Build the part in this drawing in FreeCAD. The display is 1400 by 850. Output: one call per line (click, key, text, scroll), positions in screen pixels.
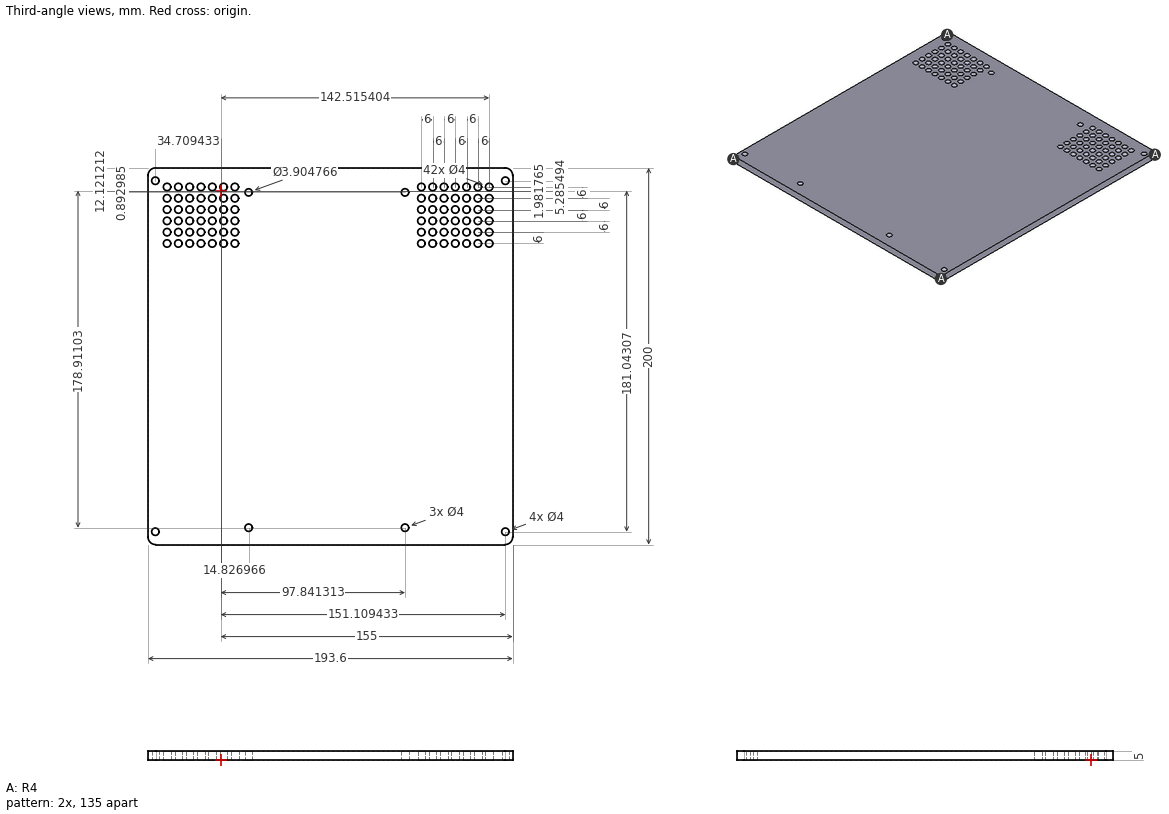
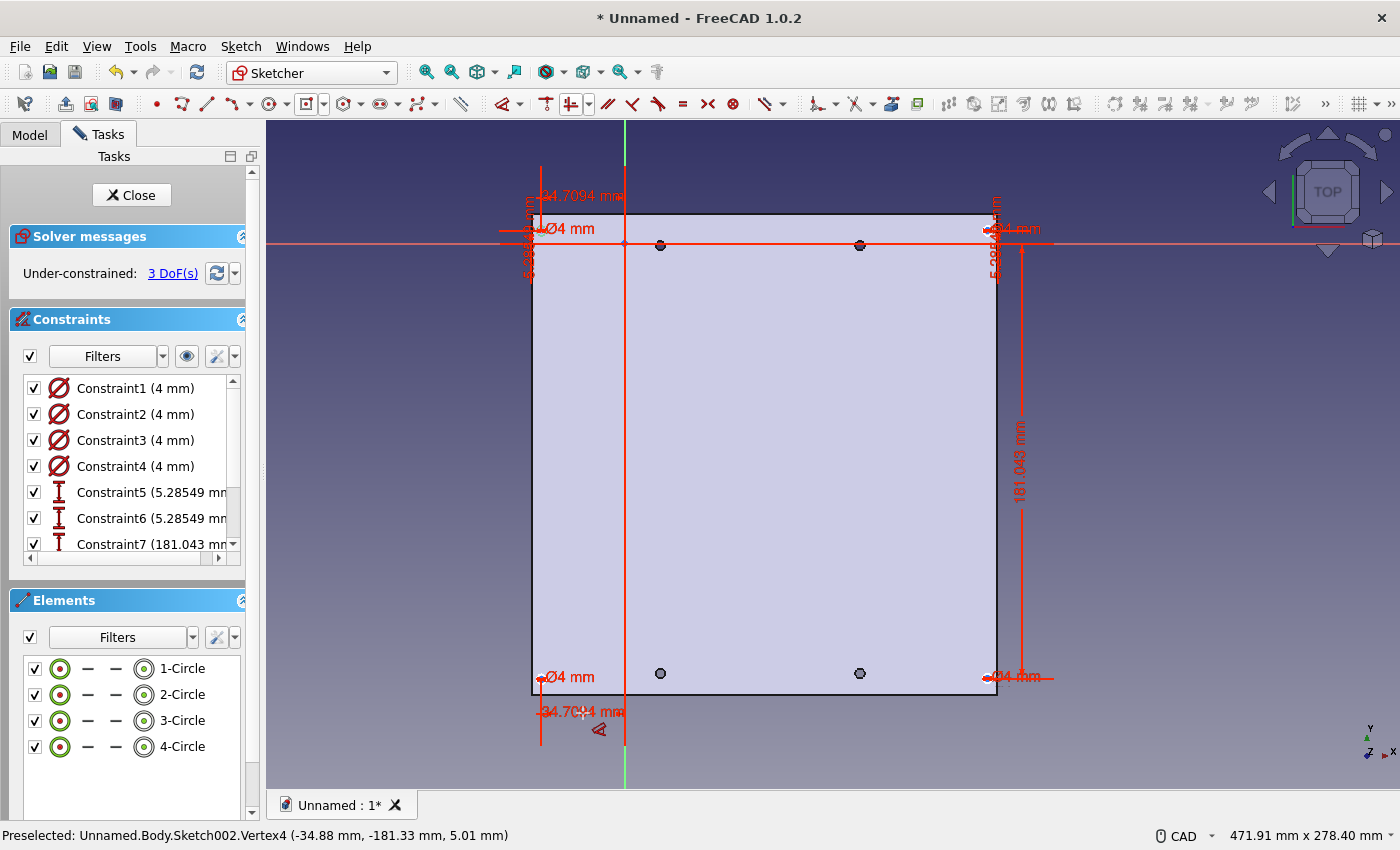
click(541, 679)
click(507, 461)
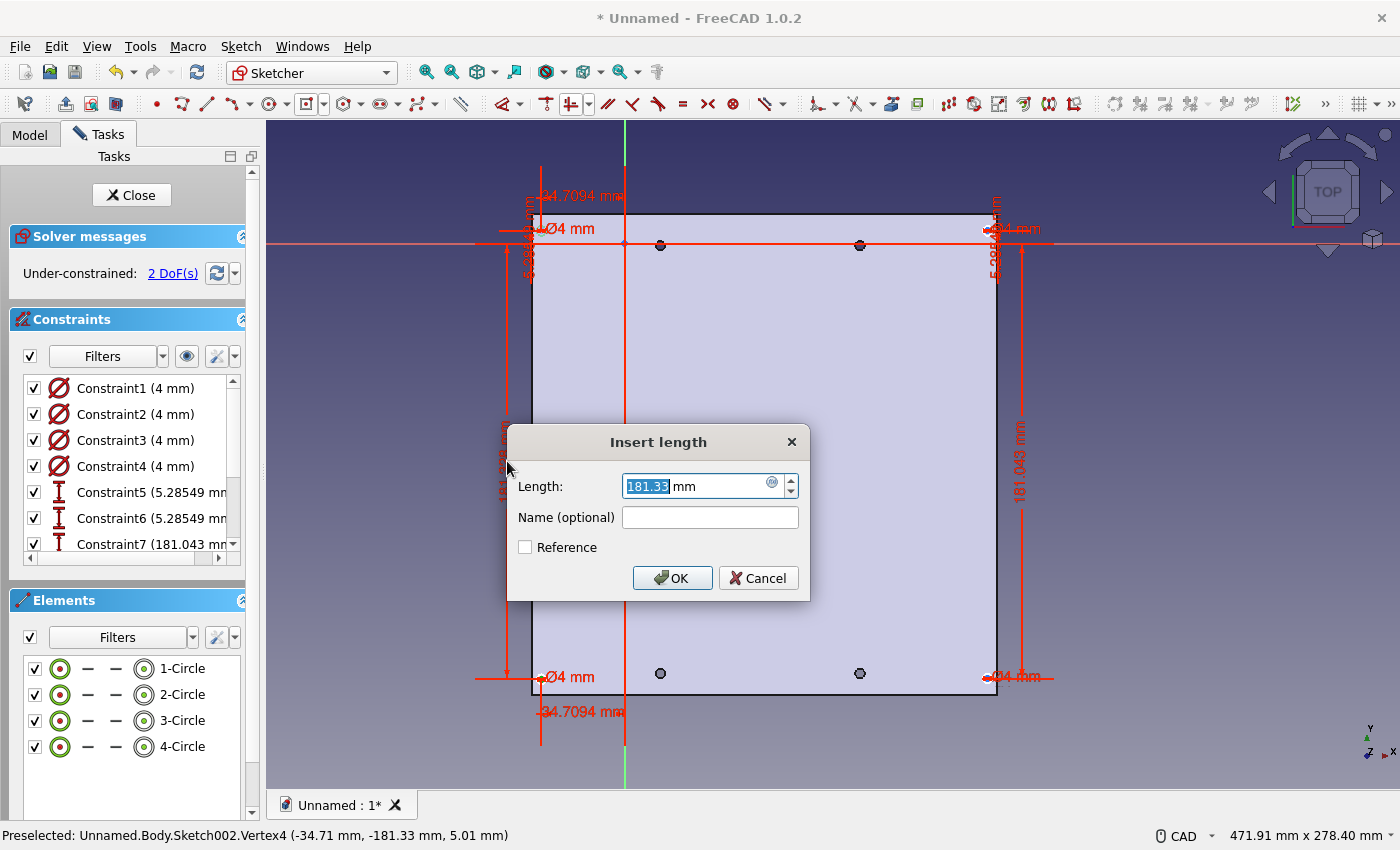
text(181.04307)
key(Return)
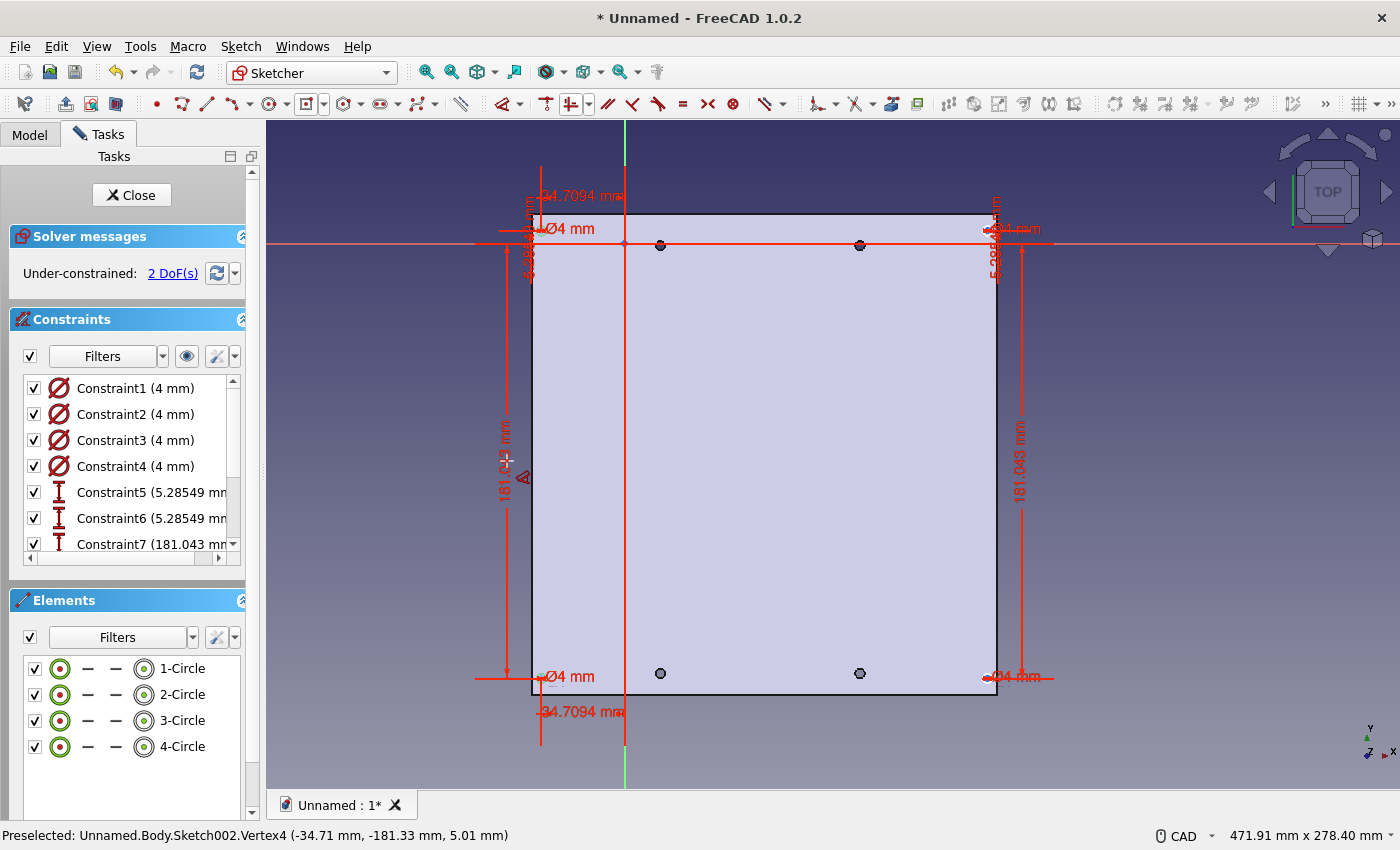
click(988, 679)
click(806, 713)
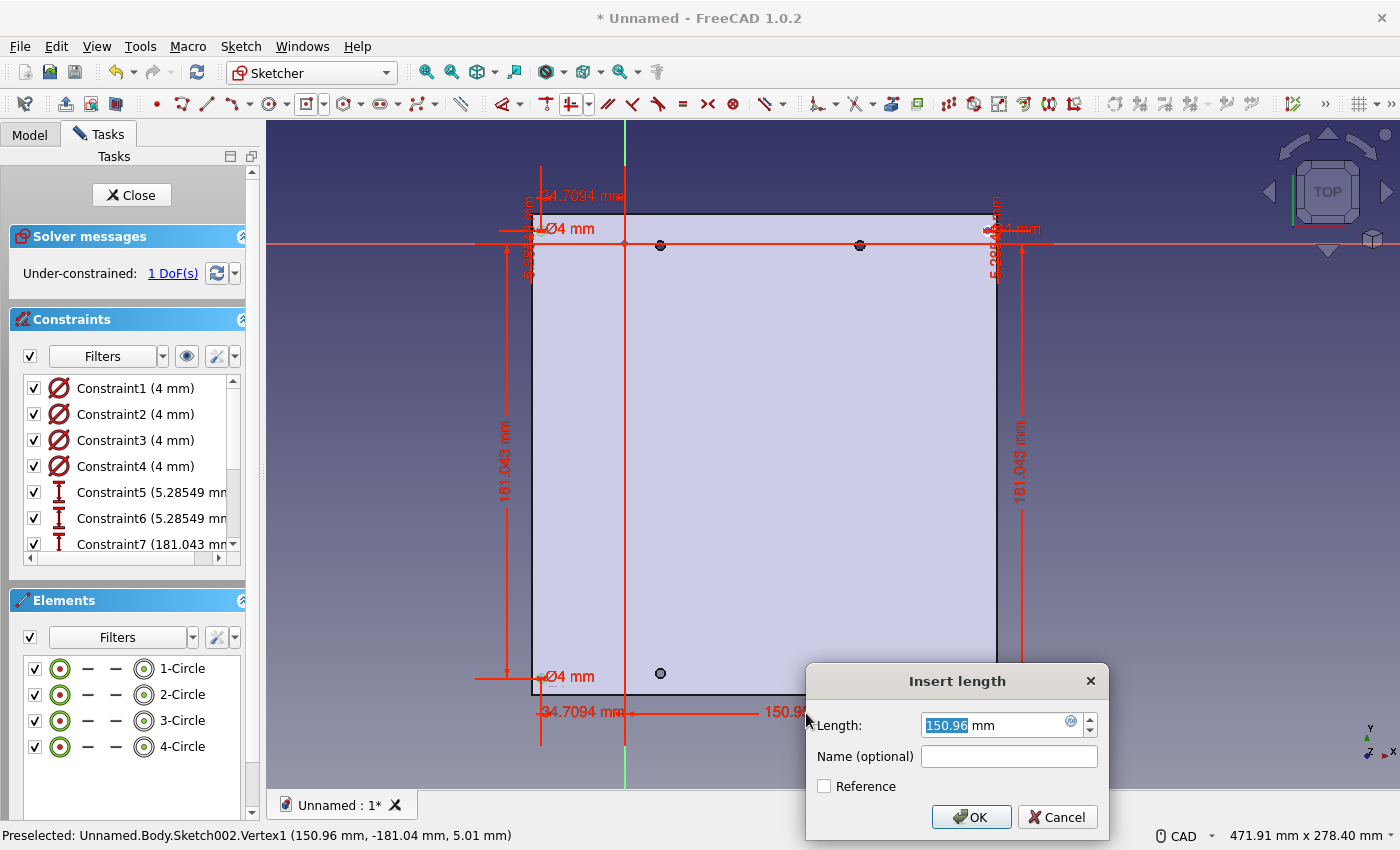
text(151.109433)
key(Return)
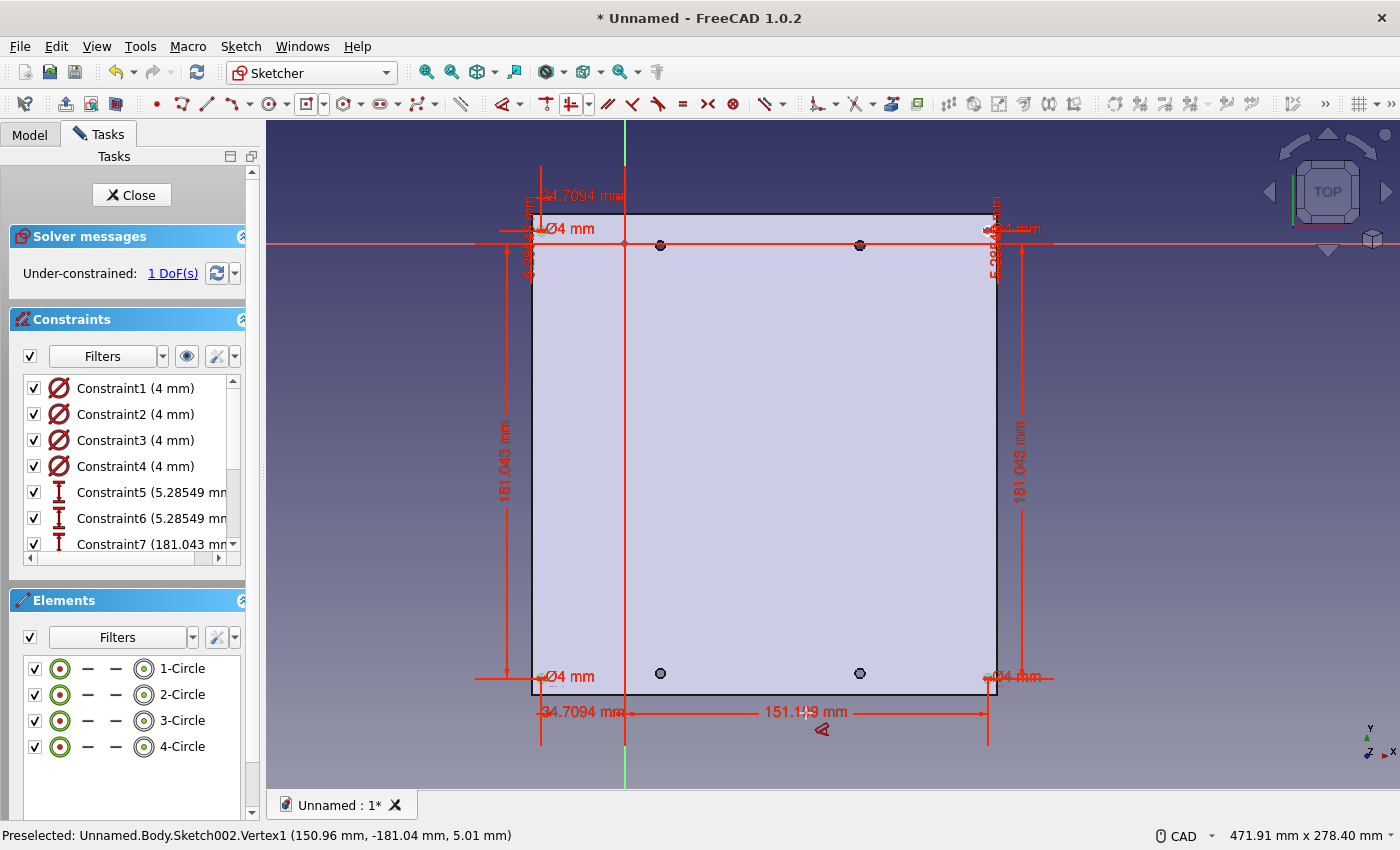
click(988, 231)
click(806, 197)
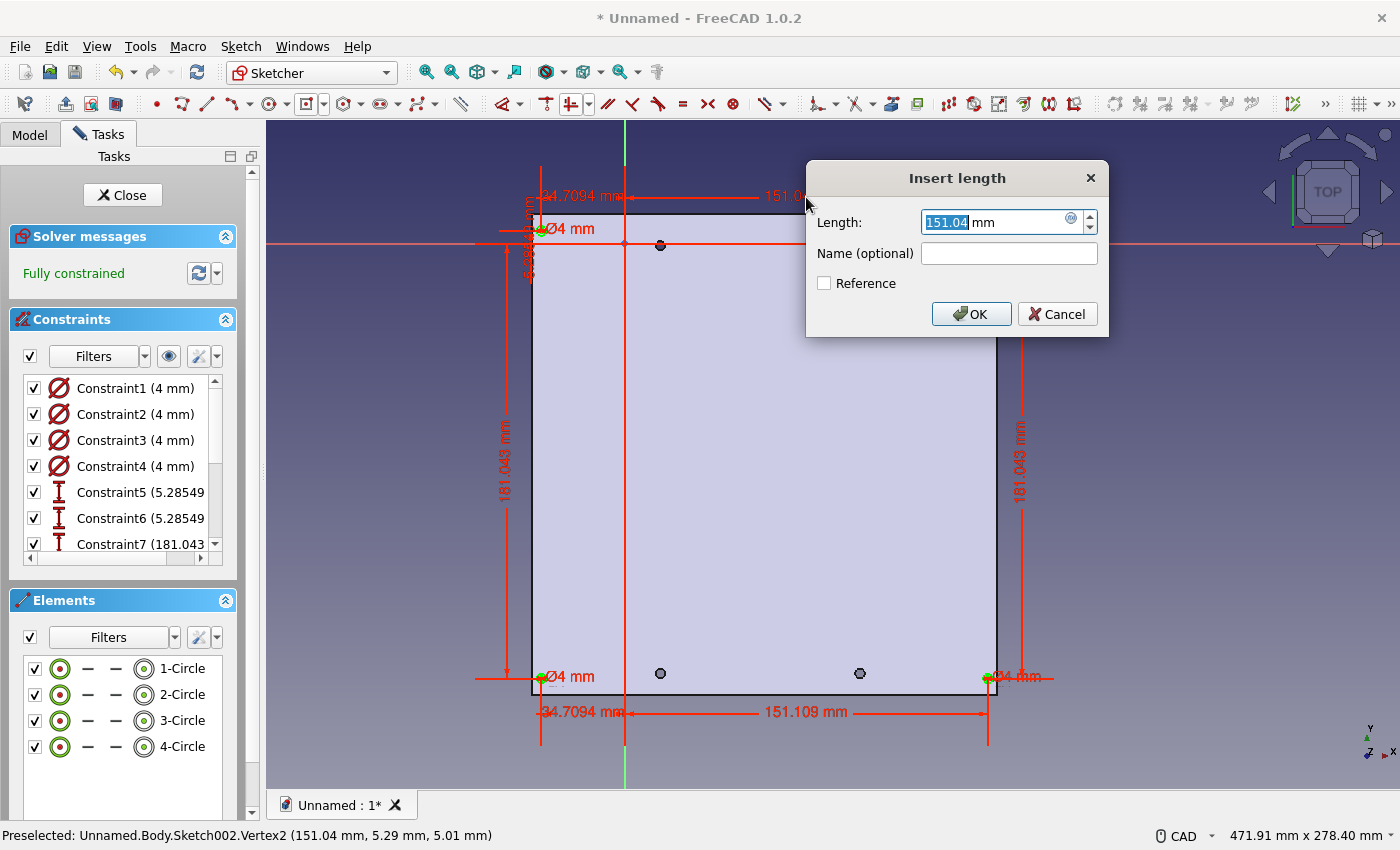
text(151.109433)
key(Return)
key(Escape)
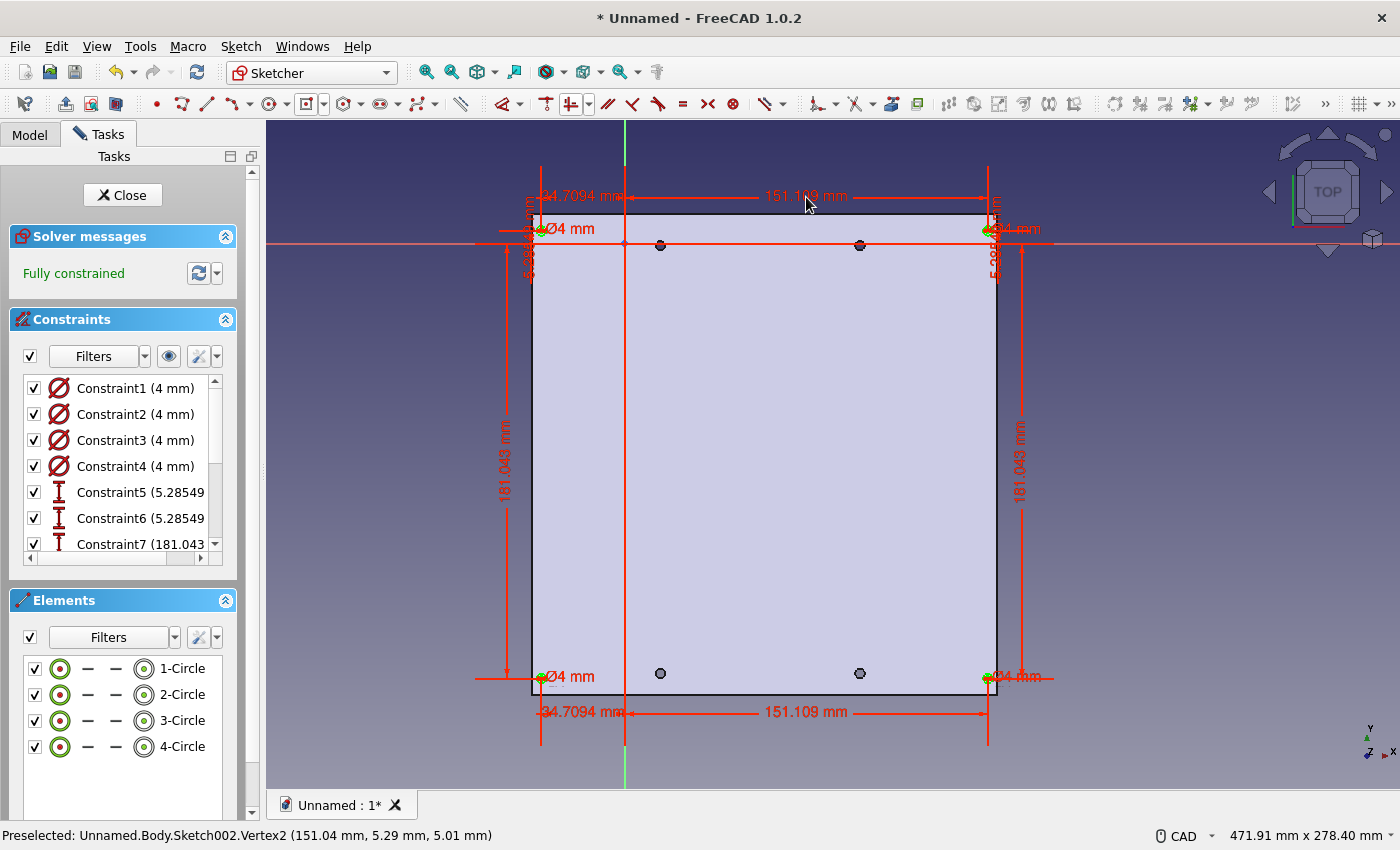
click(123, 195)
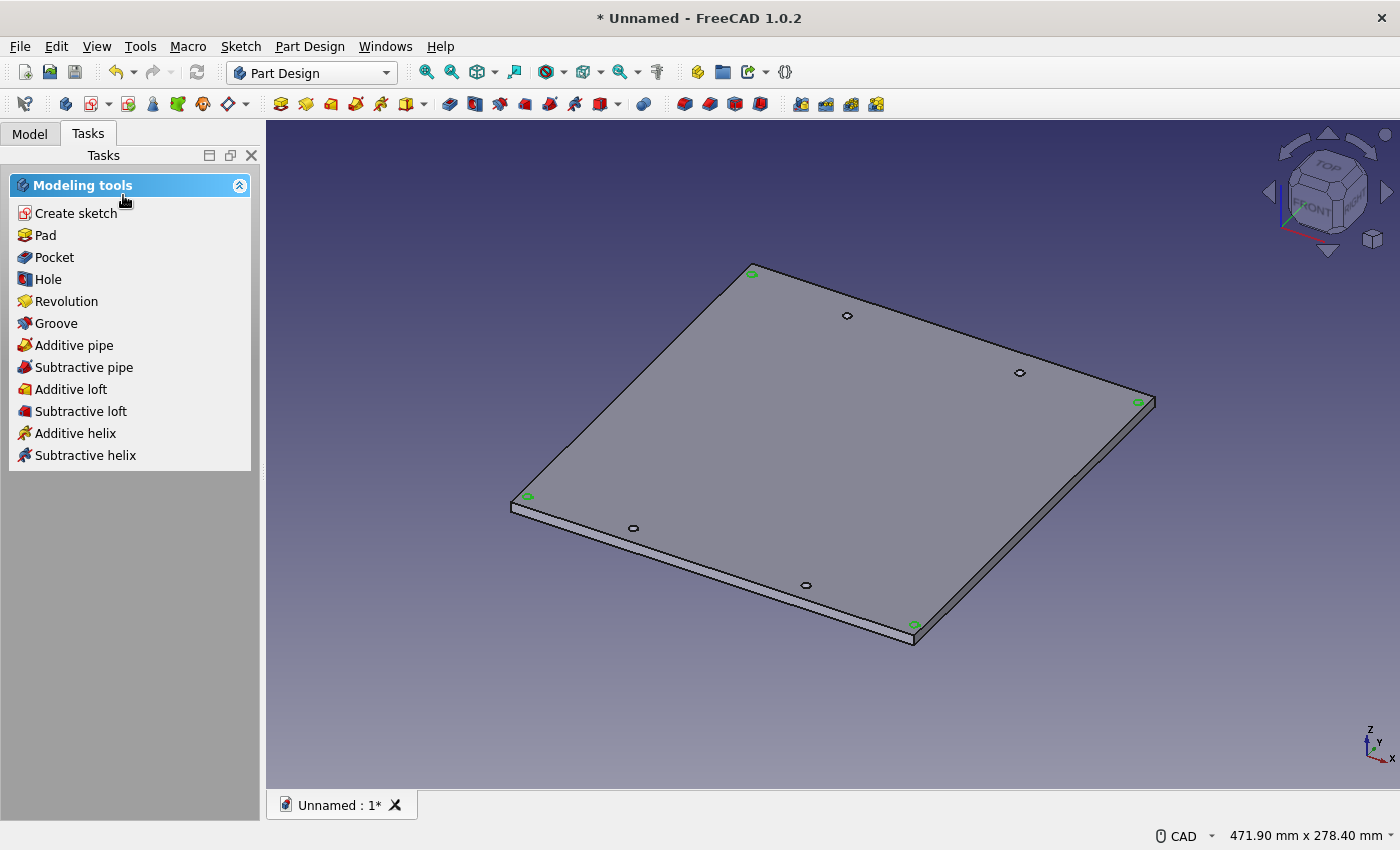
click(450, 104)